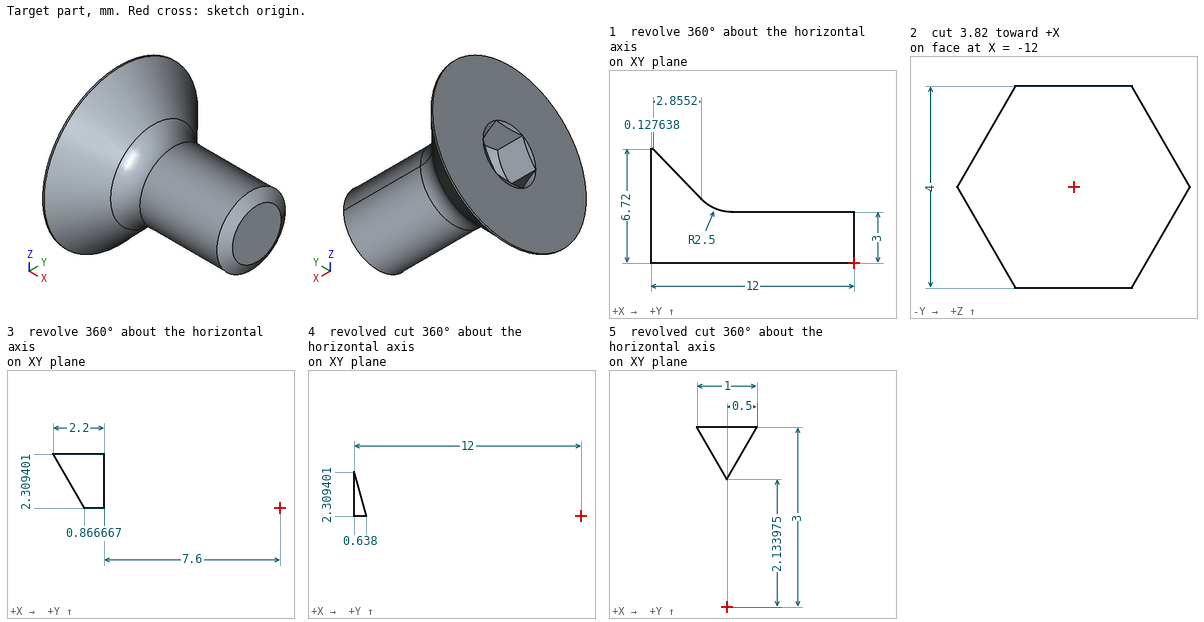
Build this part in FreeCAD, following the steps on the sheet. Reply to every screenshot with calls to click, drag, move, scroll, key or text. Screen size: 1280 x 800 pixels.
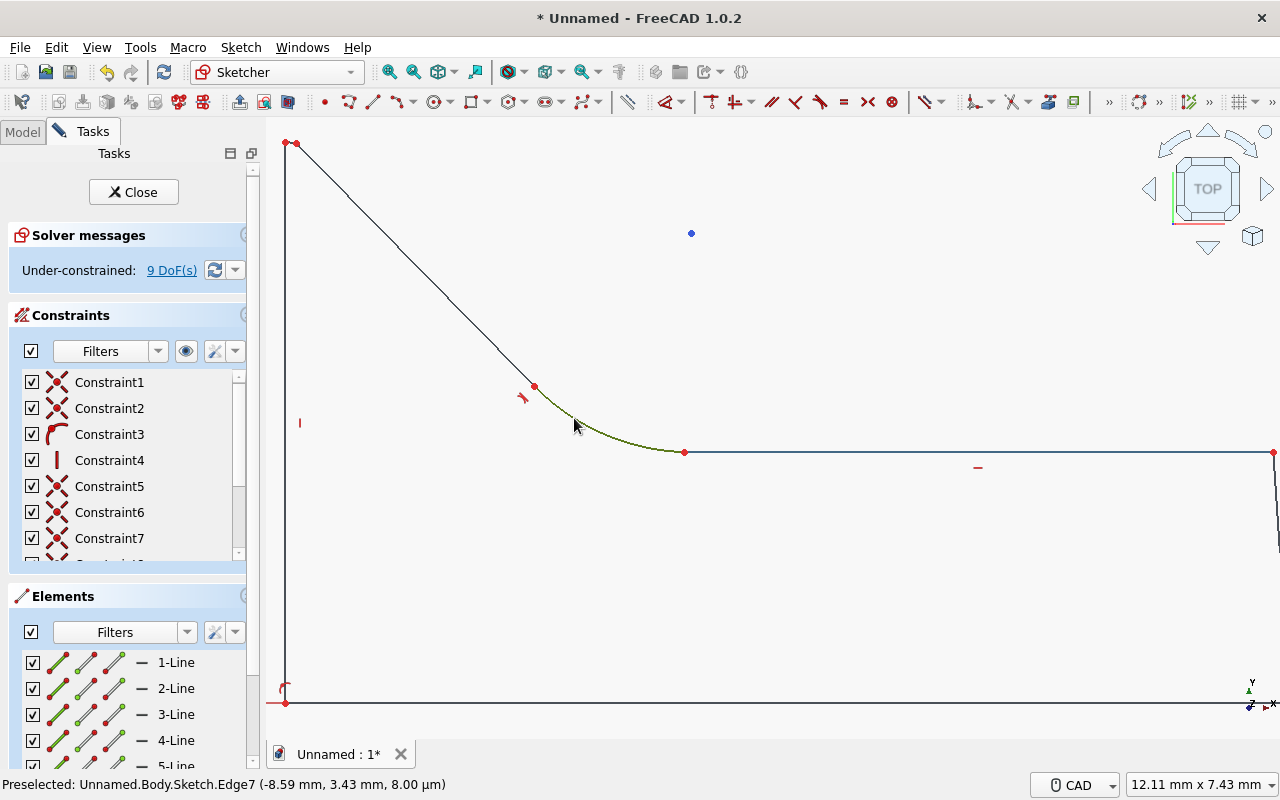
key(t)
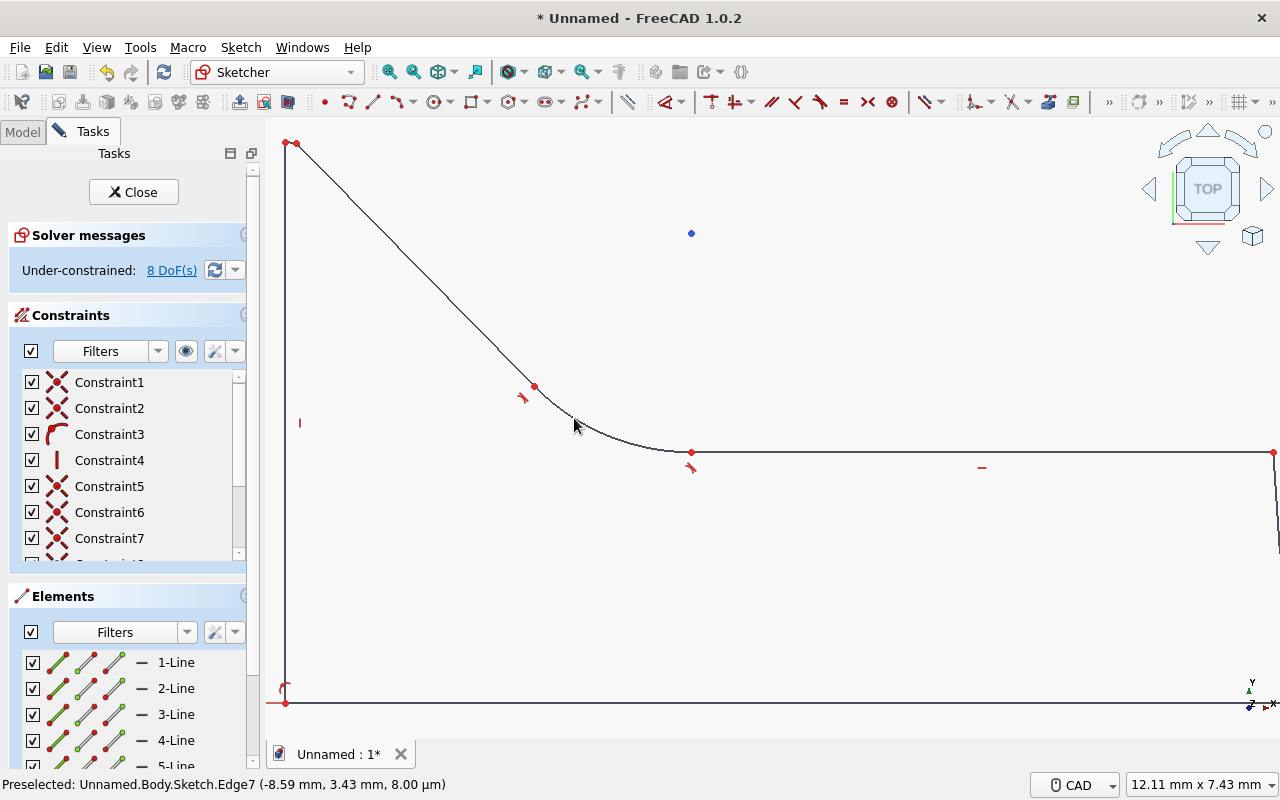
scroll(604, 436, down, 3)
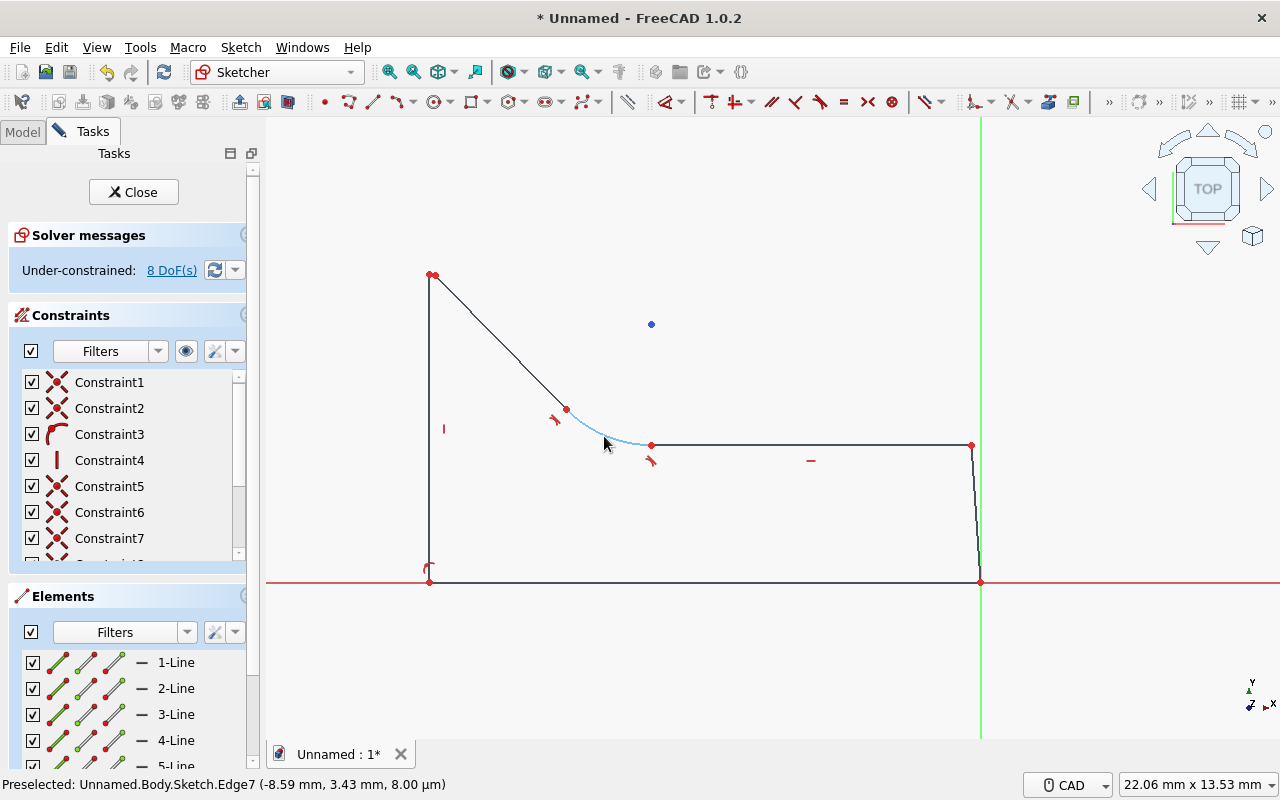
scroll(432, 275, up, 8)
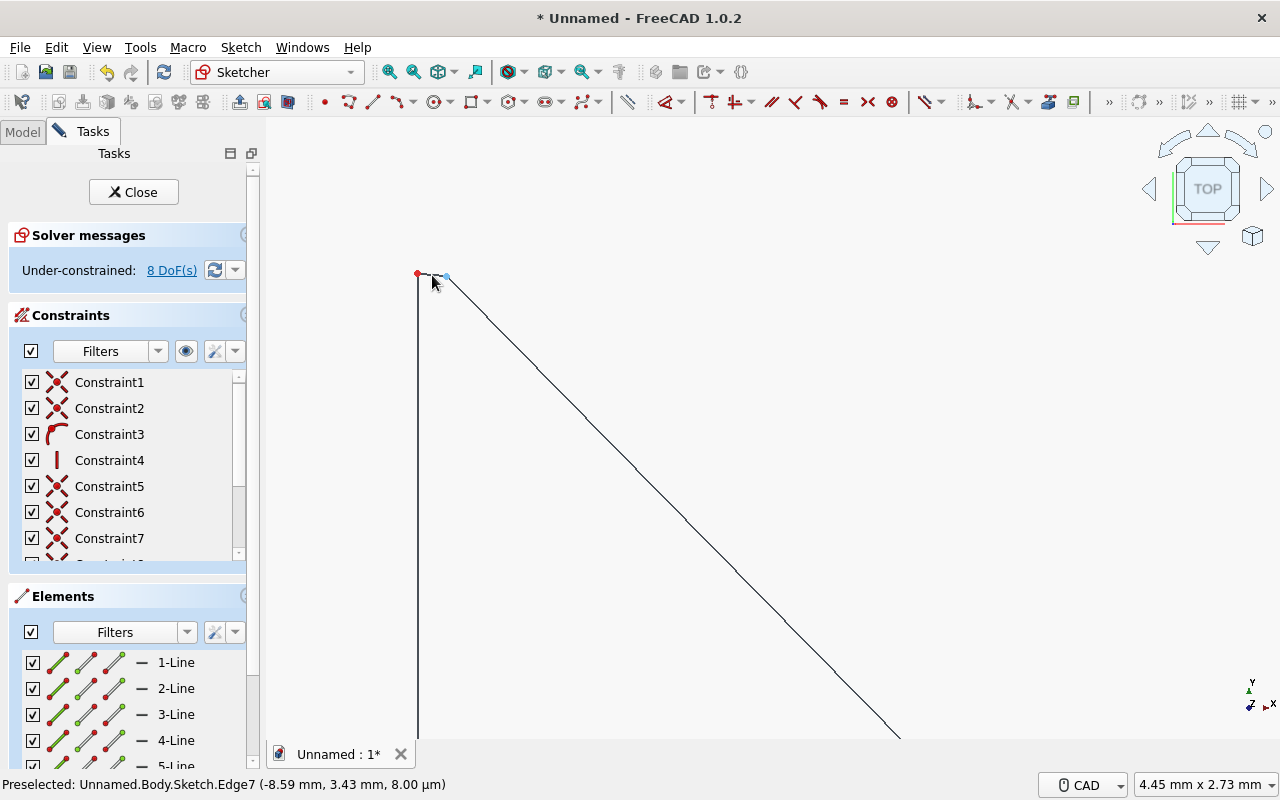
click(432, 275)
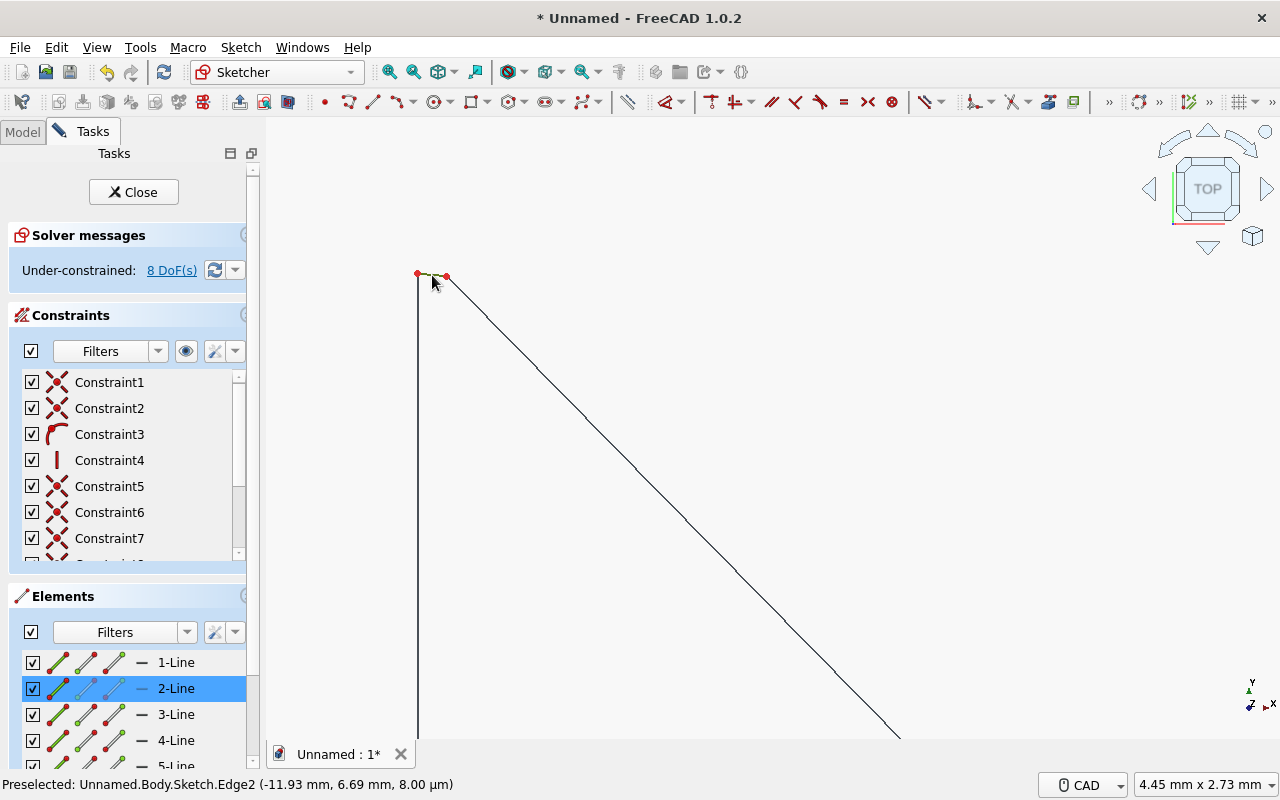
key(h)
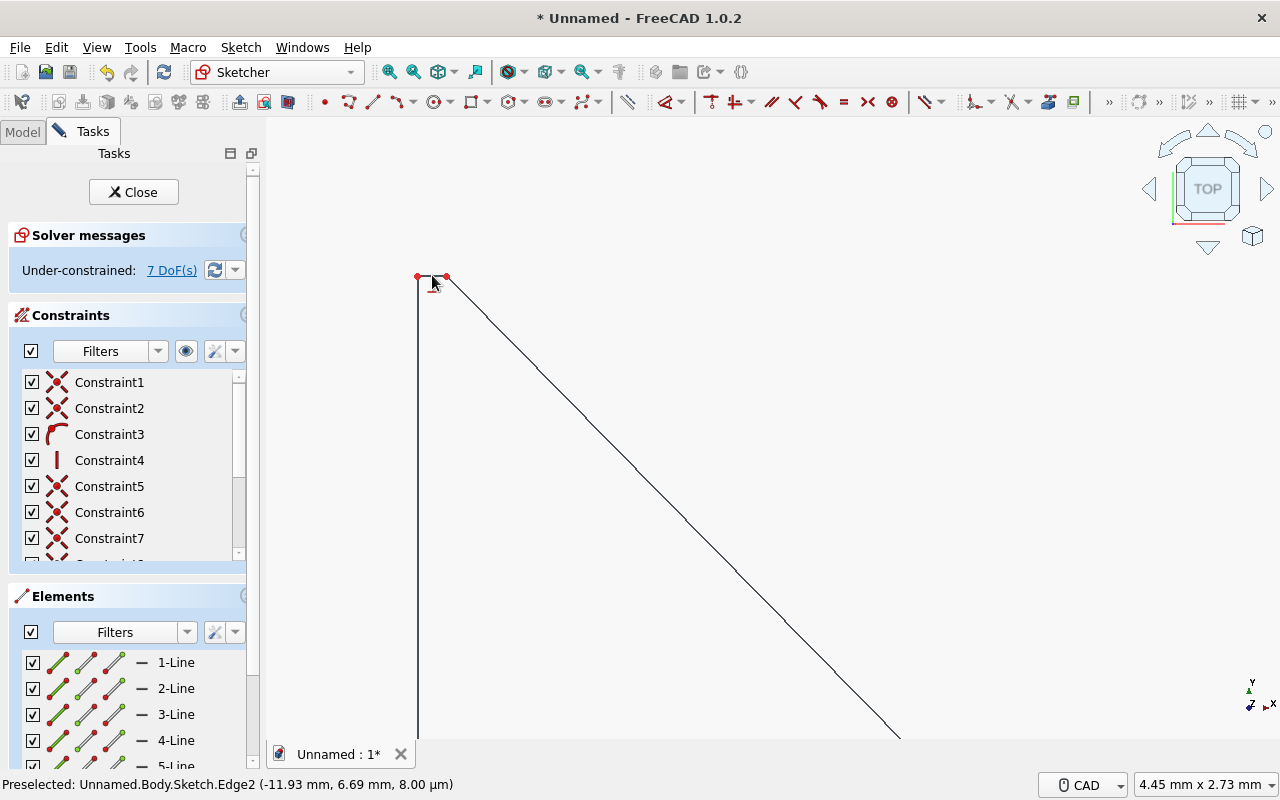
scroll(432, 275, down, 8)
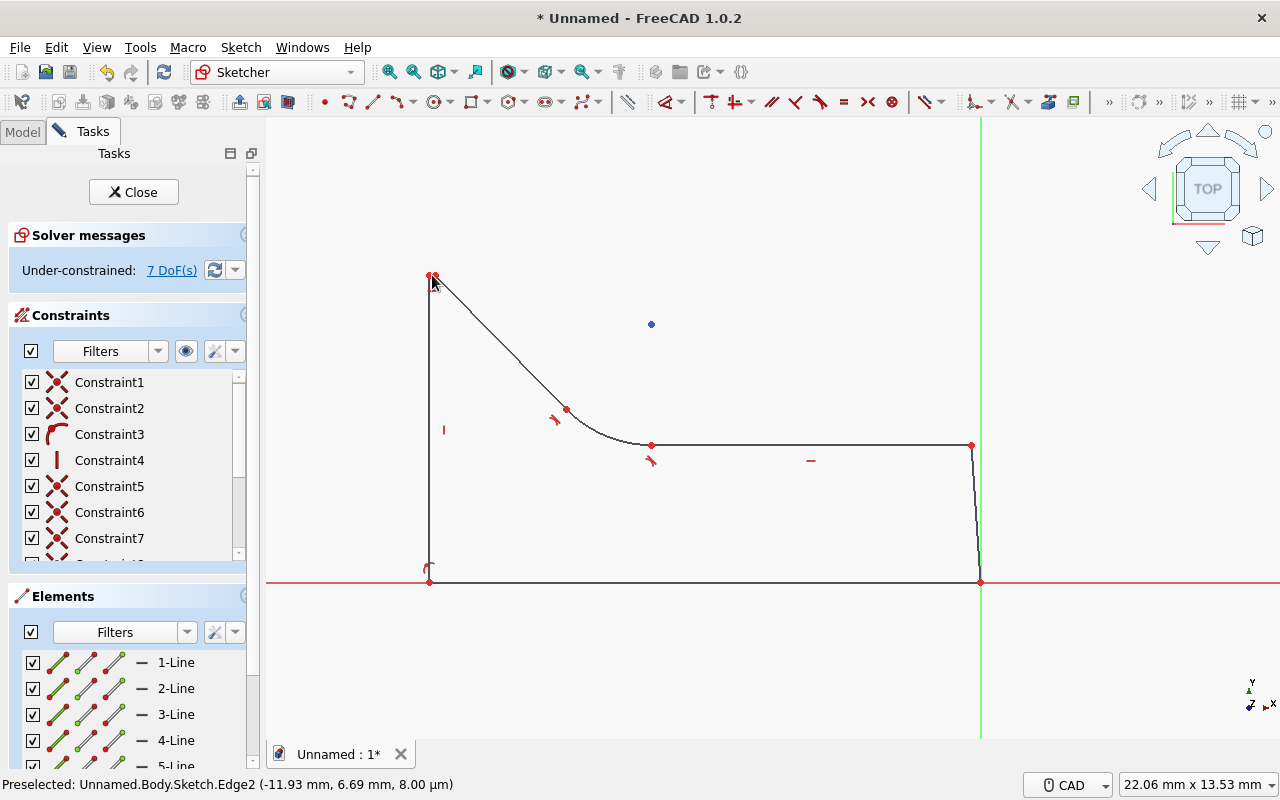
scroll(978, 541, up, 9)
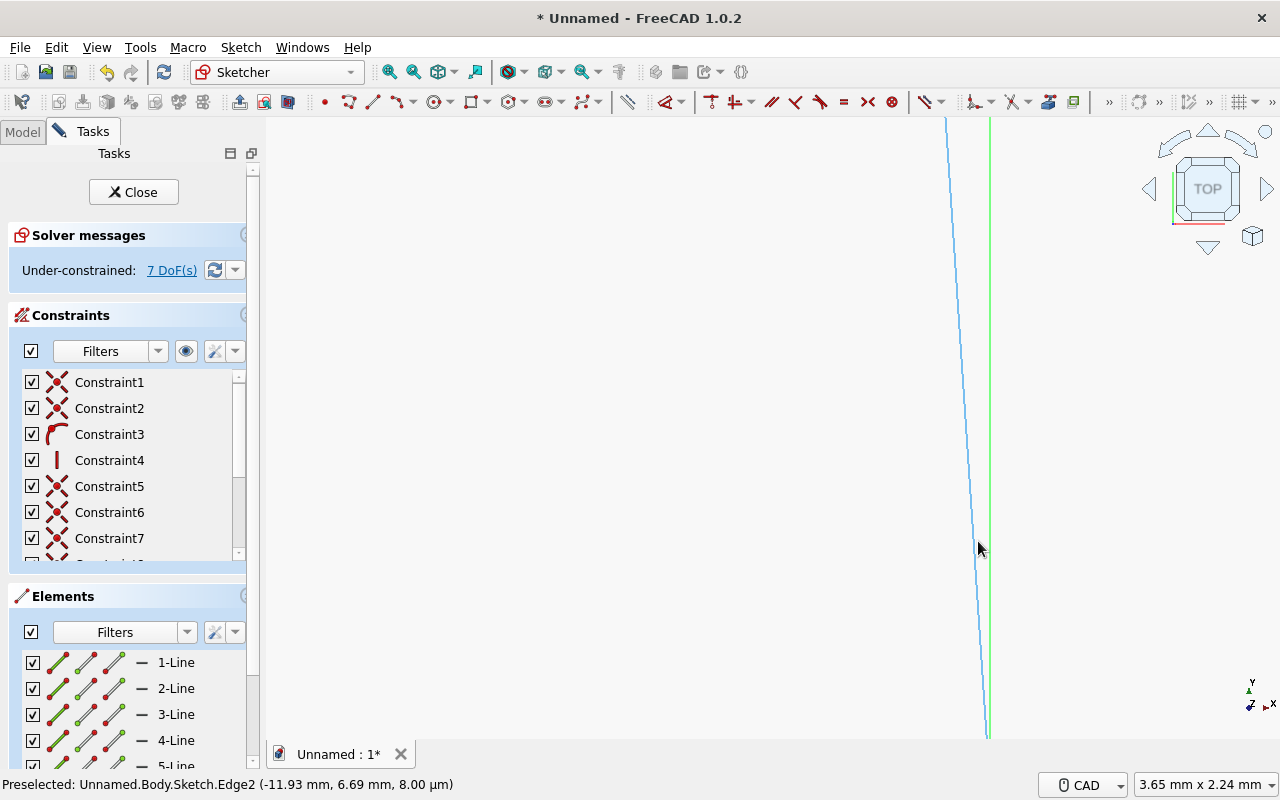
click(974, 541)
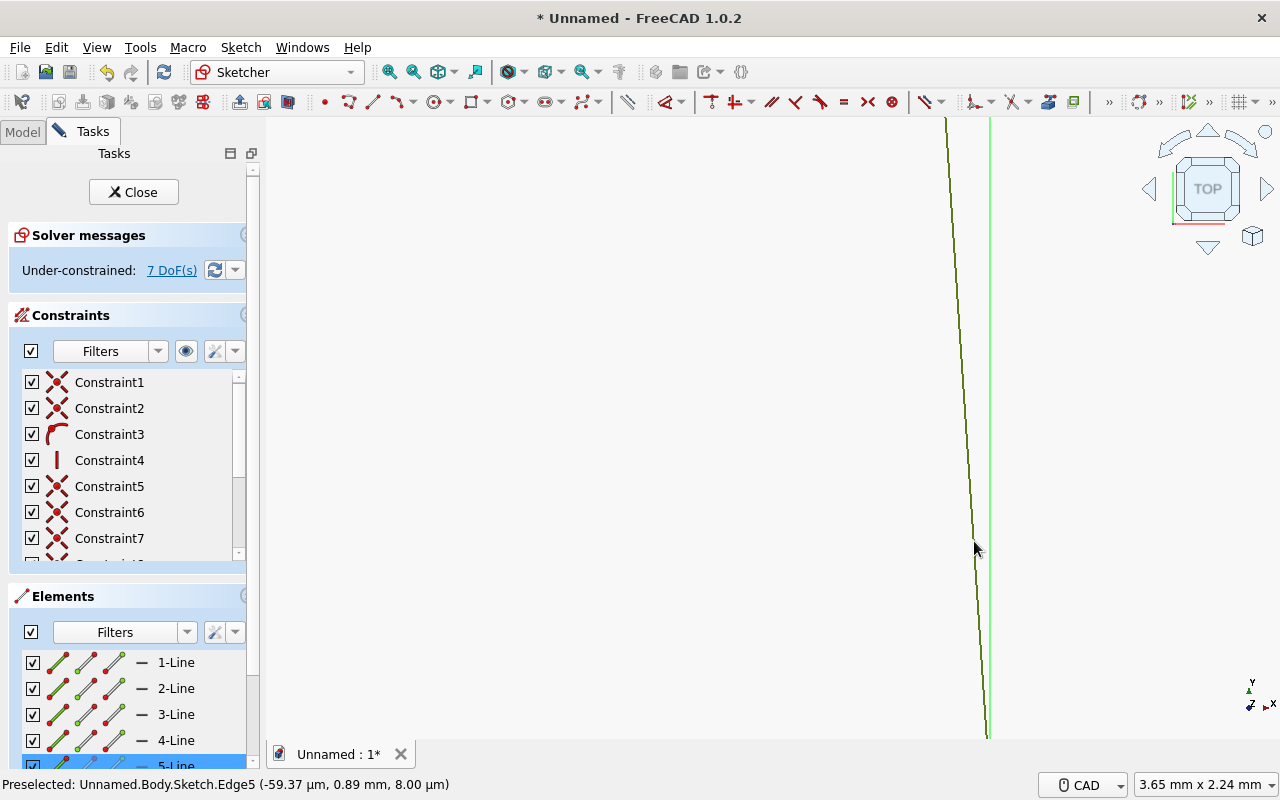
click(754, 102)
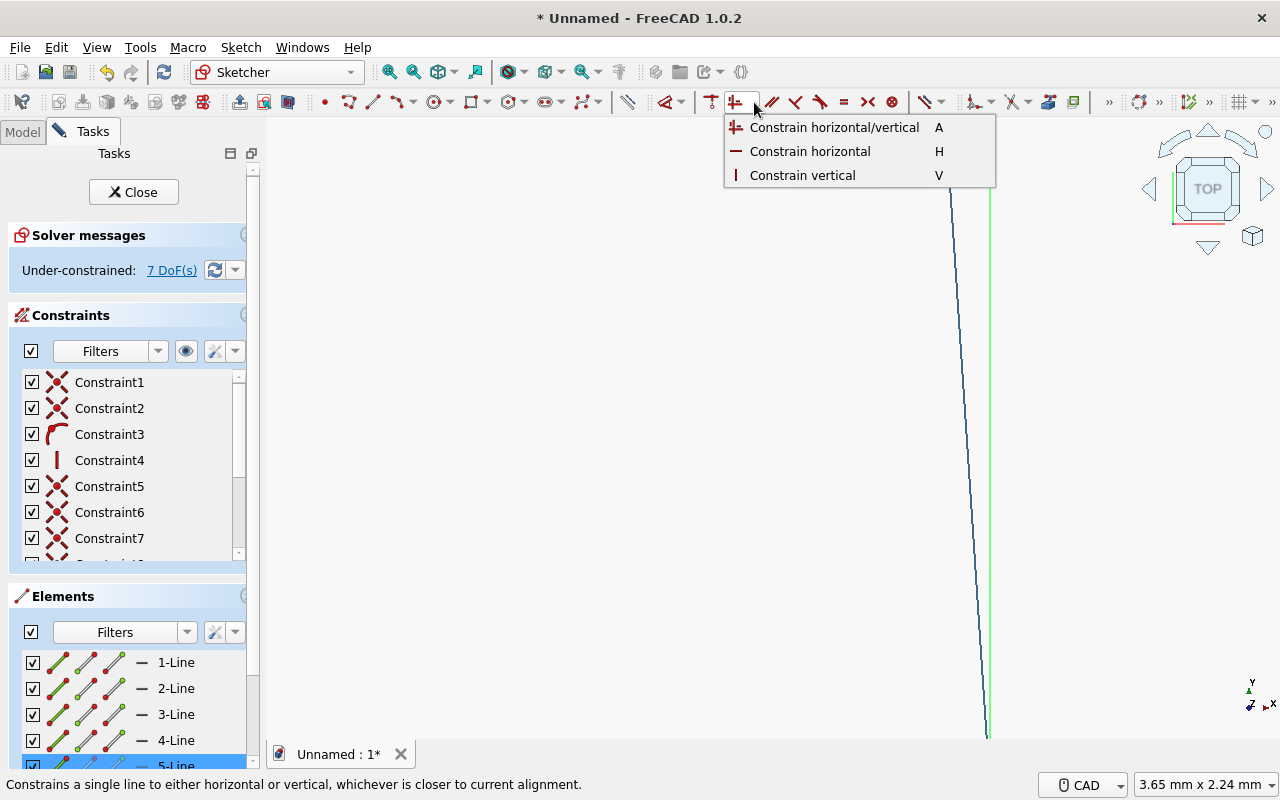
click(860, 175)